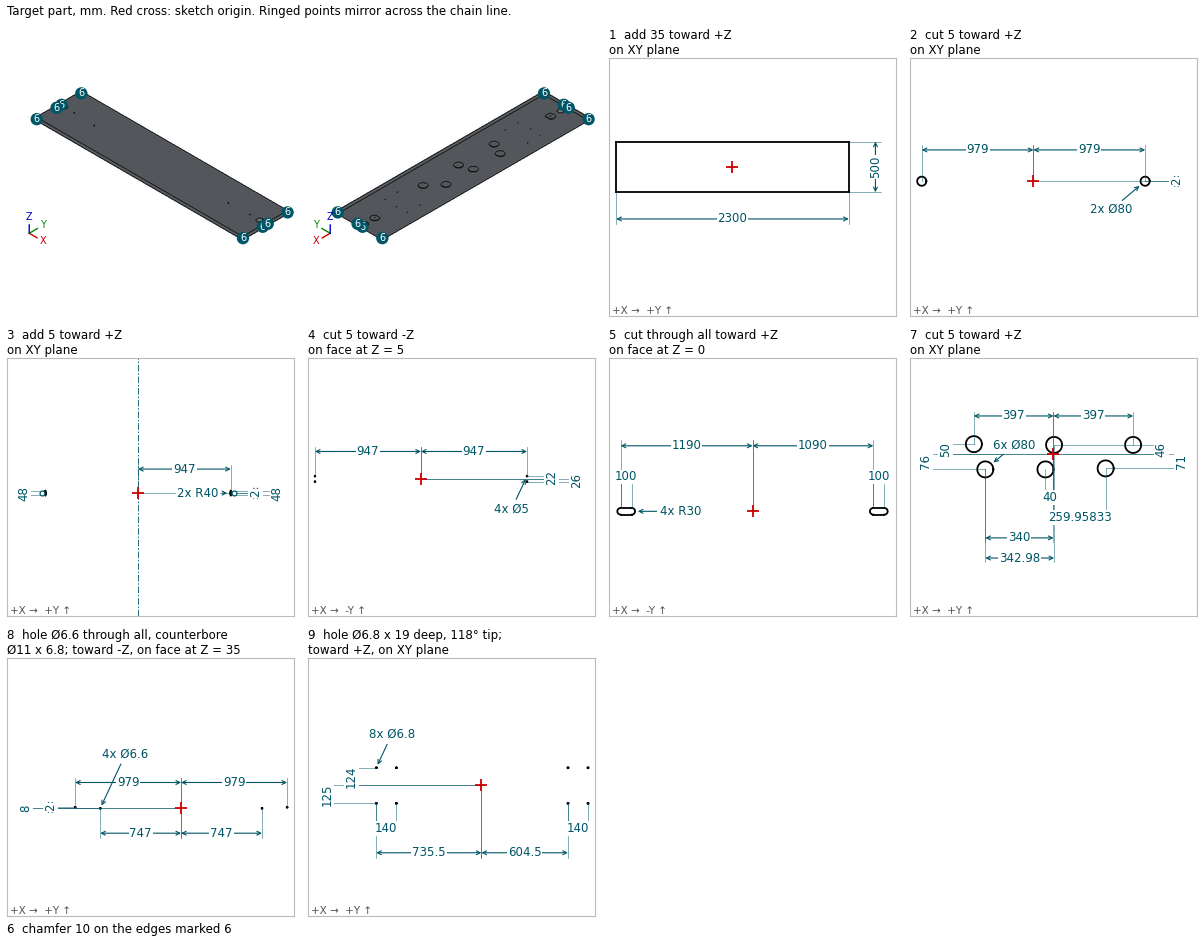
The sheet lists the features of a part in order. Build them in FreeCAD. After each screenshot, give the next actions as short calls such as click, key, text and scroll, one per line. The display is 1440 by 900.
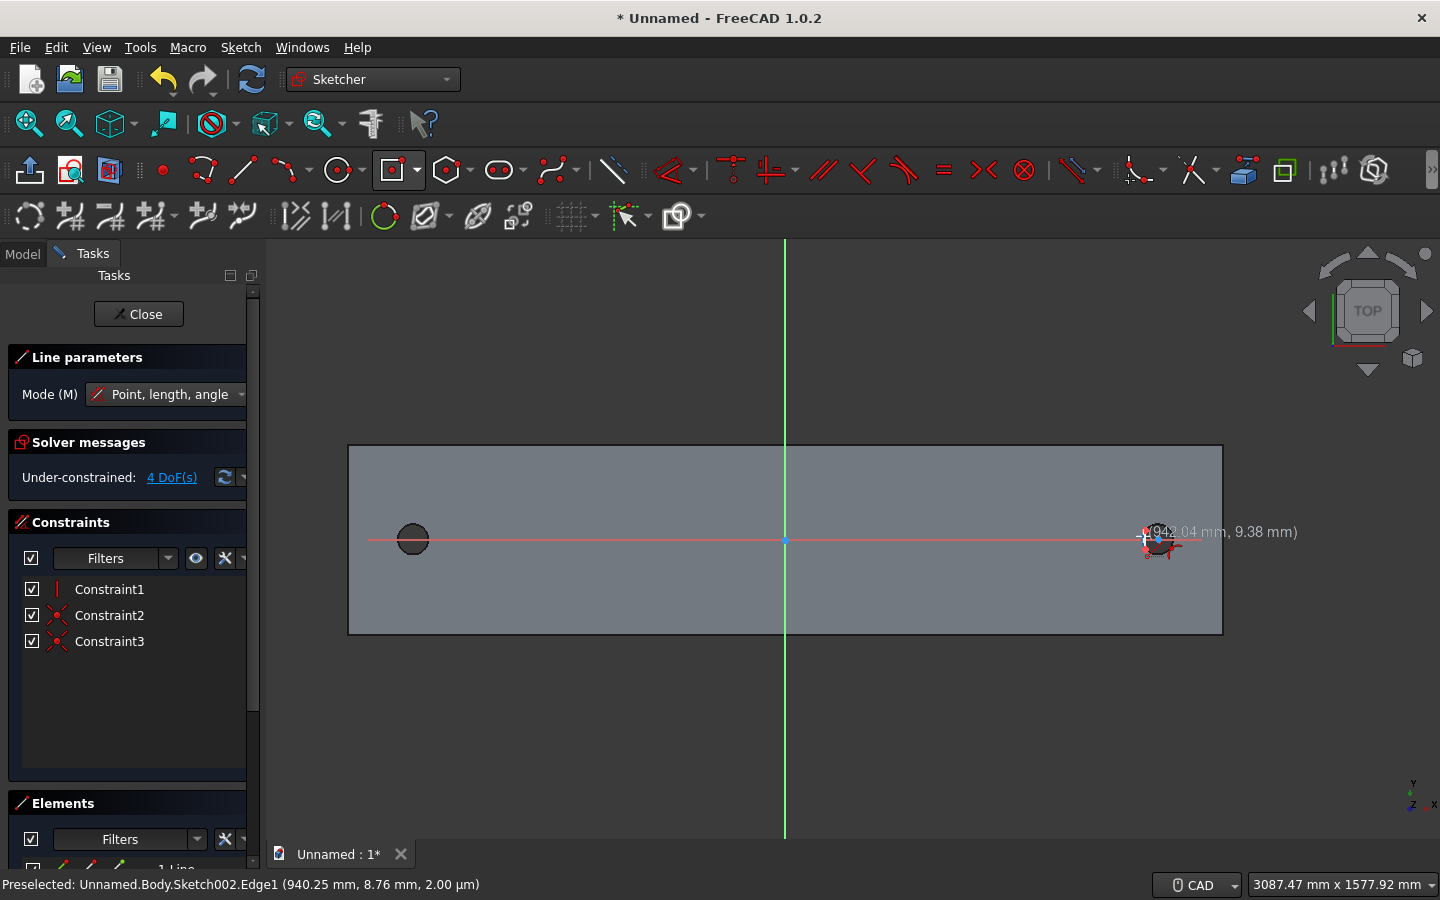
scroll(425, 549, up, 4)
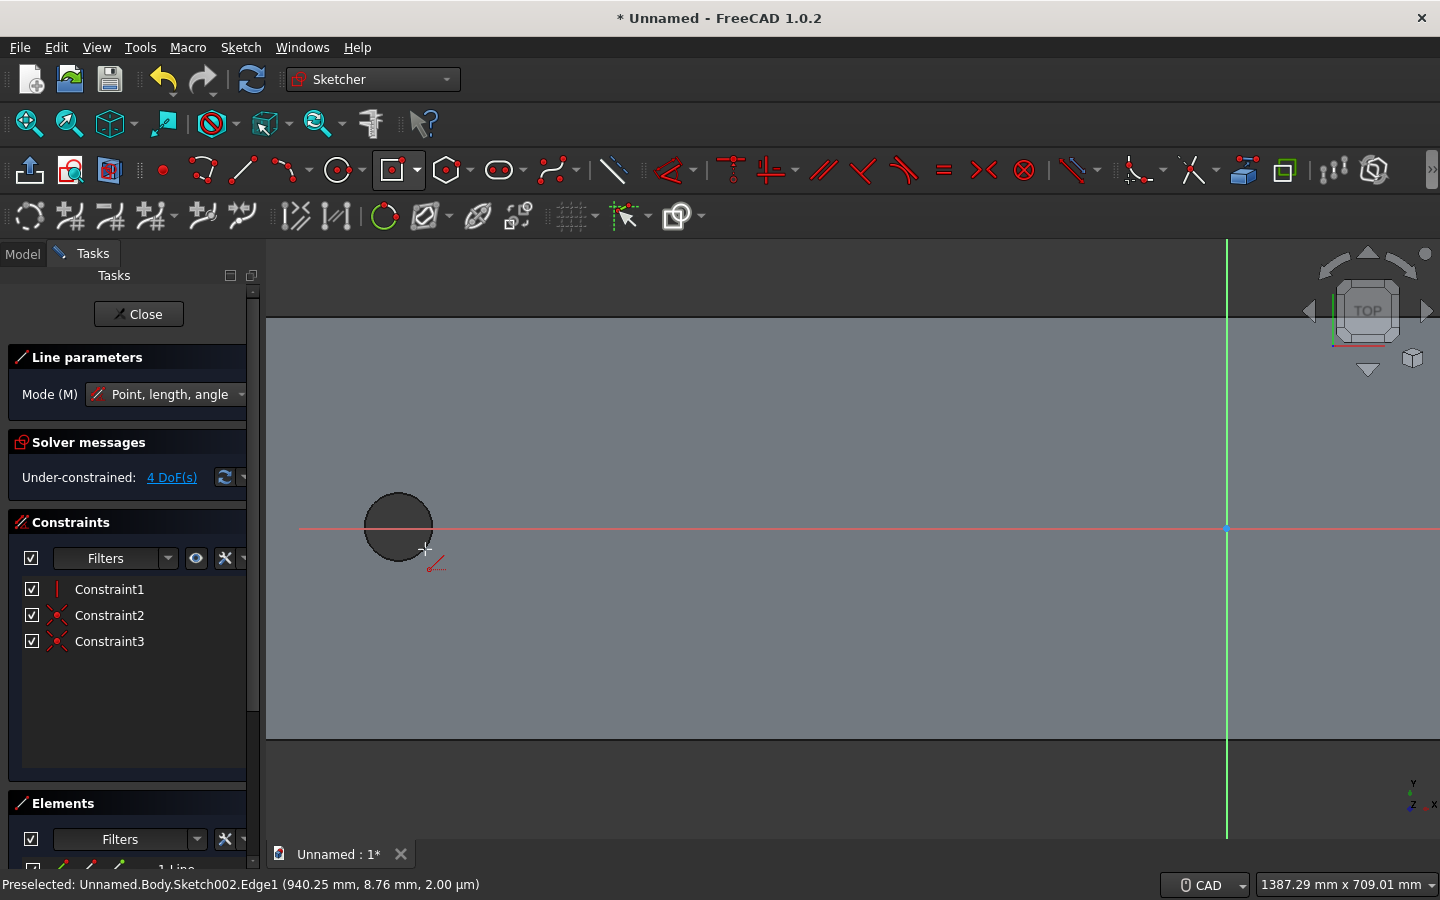
click(426, 547)
click(426, 507)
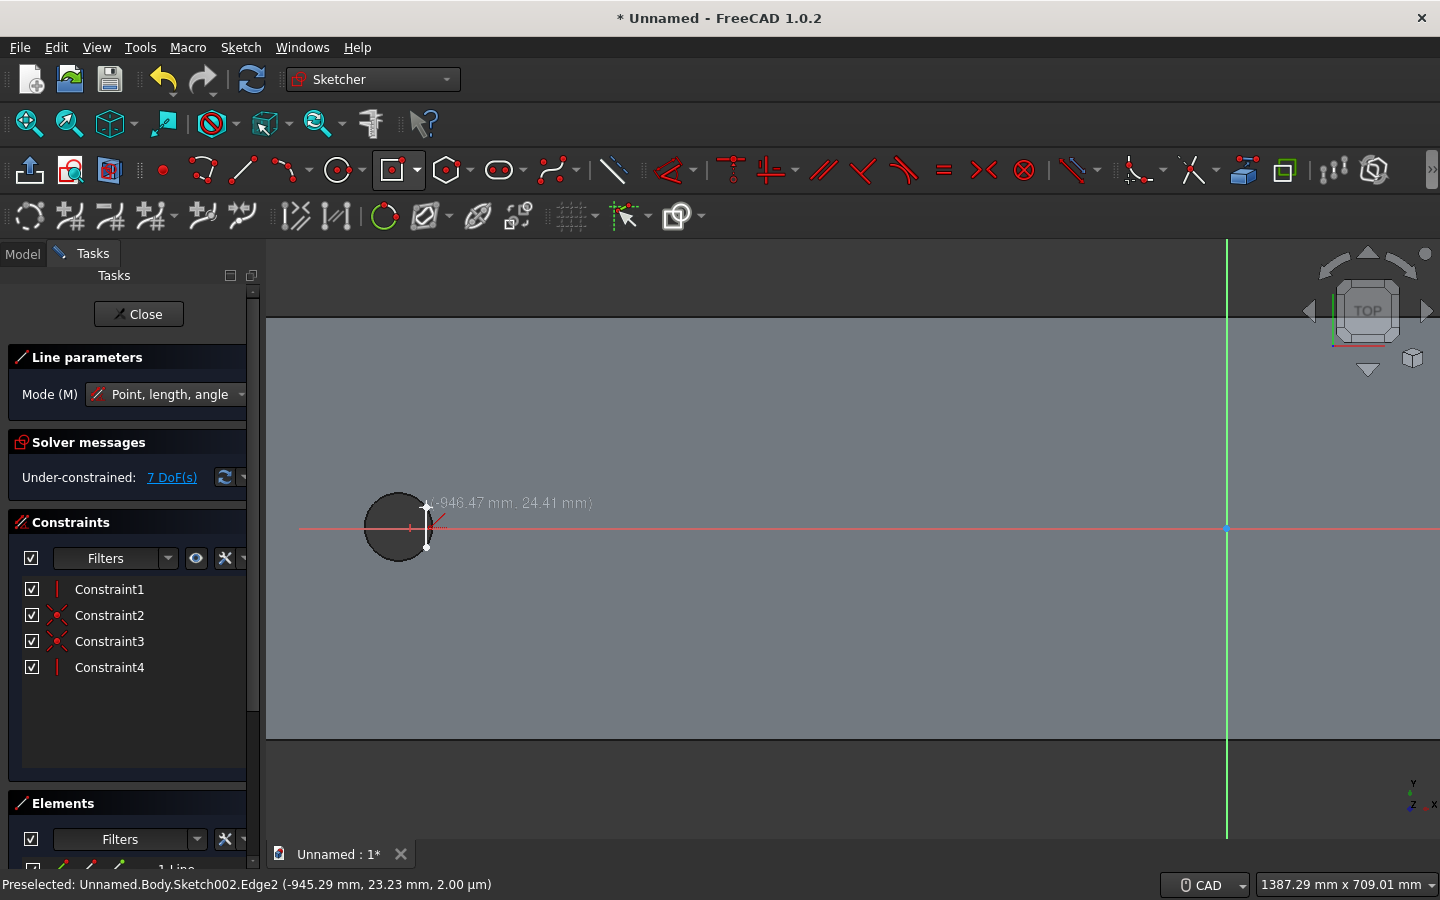
click(284, 170)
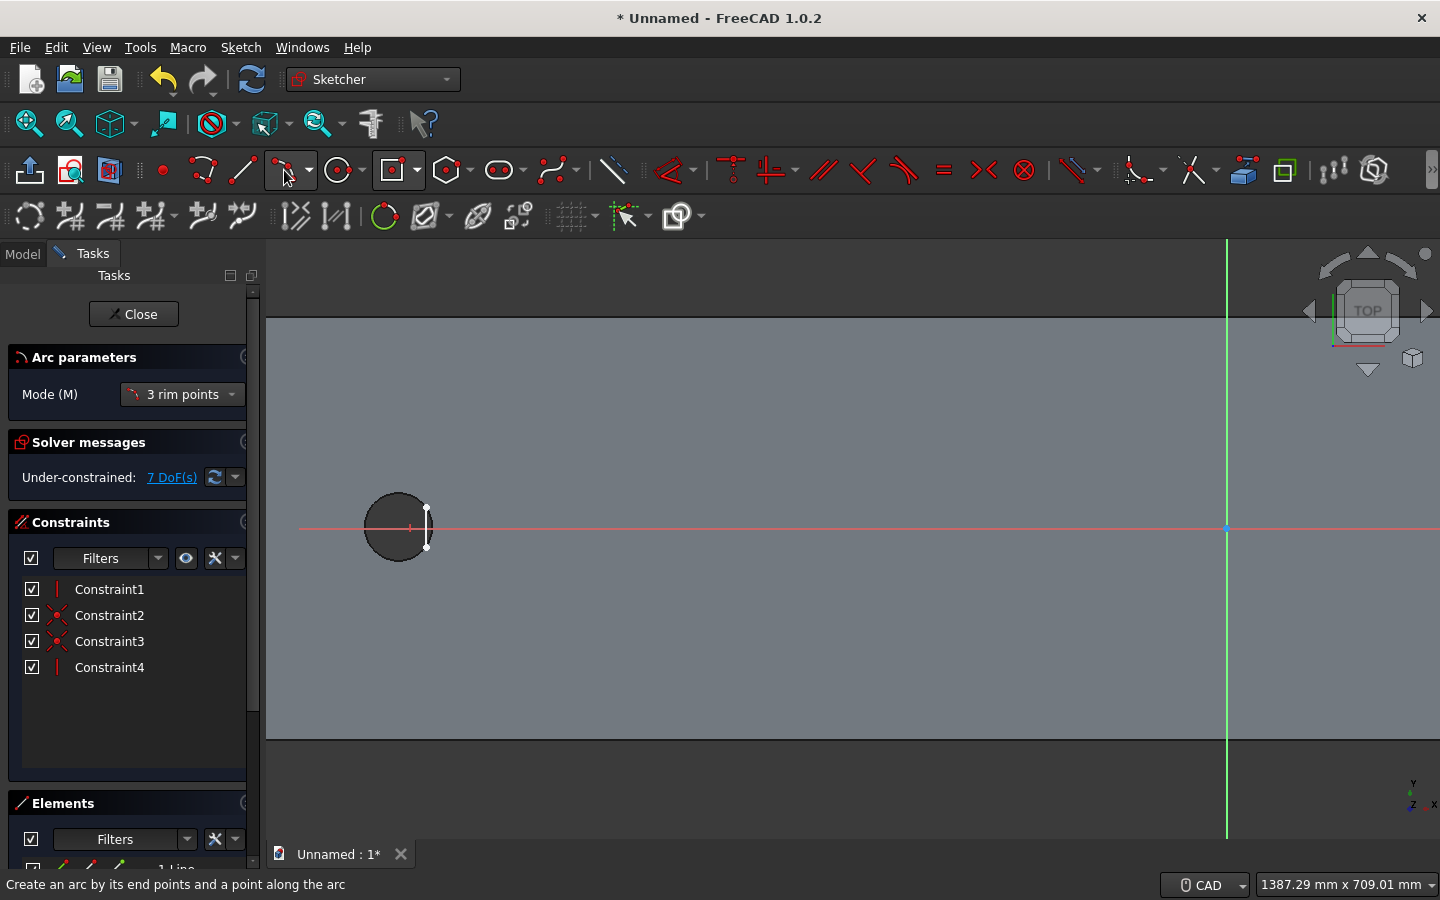
click(426, 508)
click(426, 548)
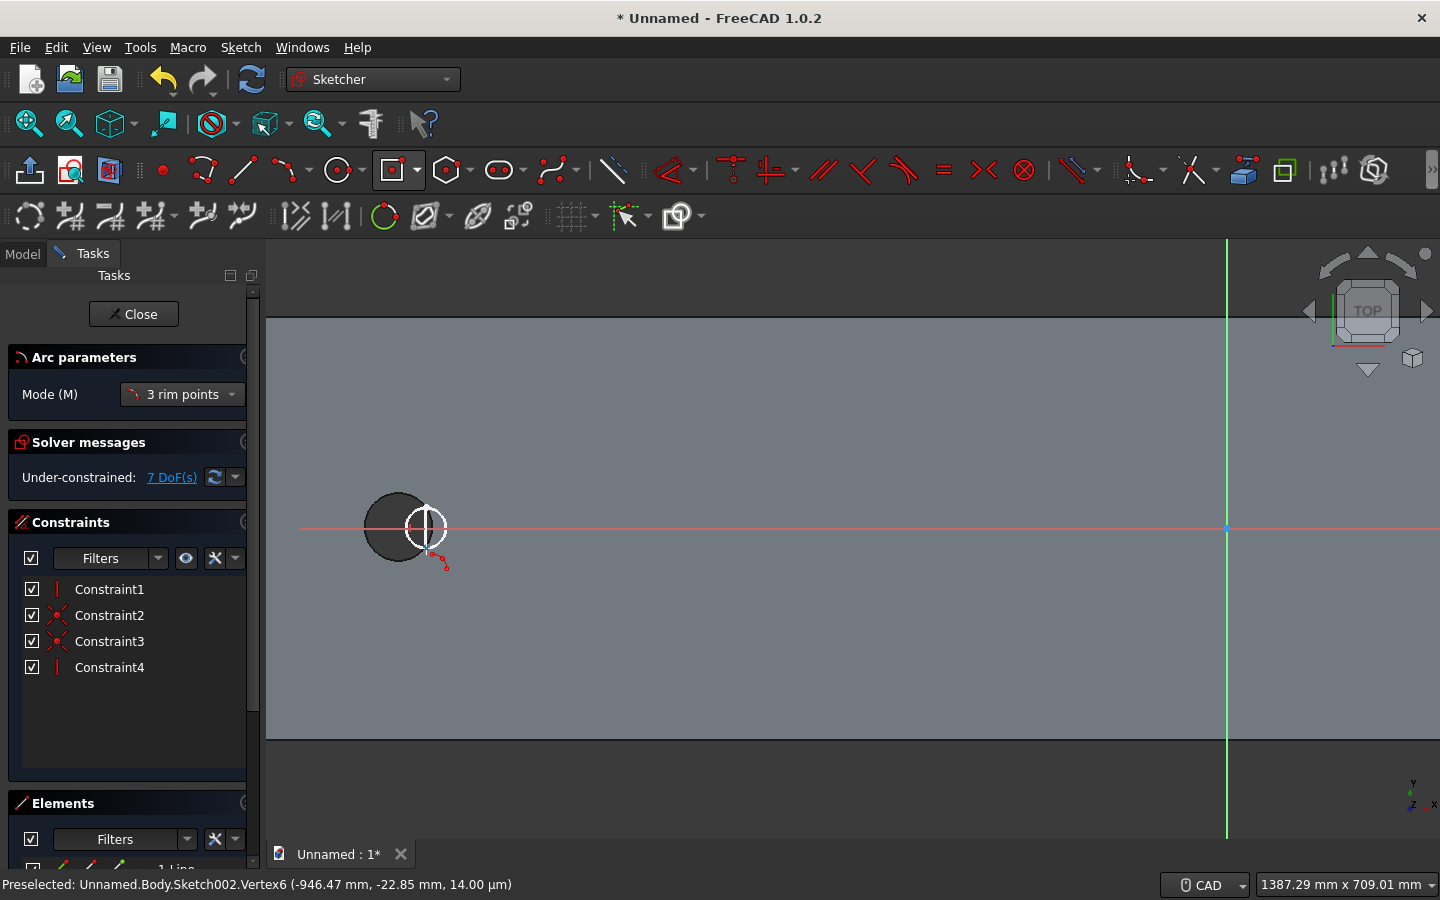
scroll(432, 523, up, 5)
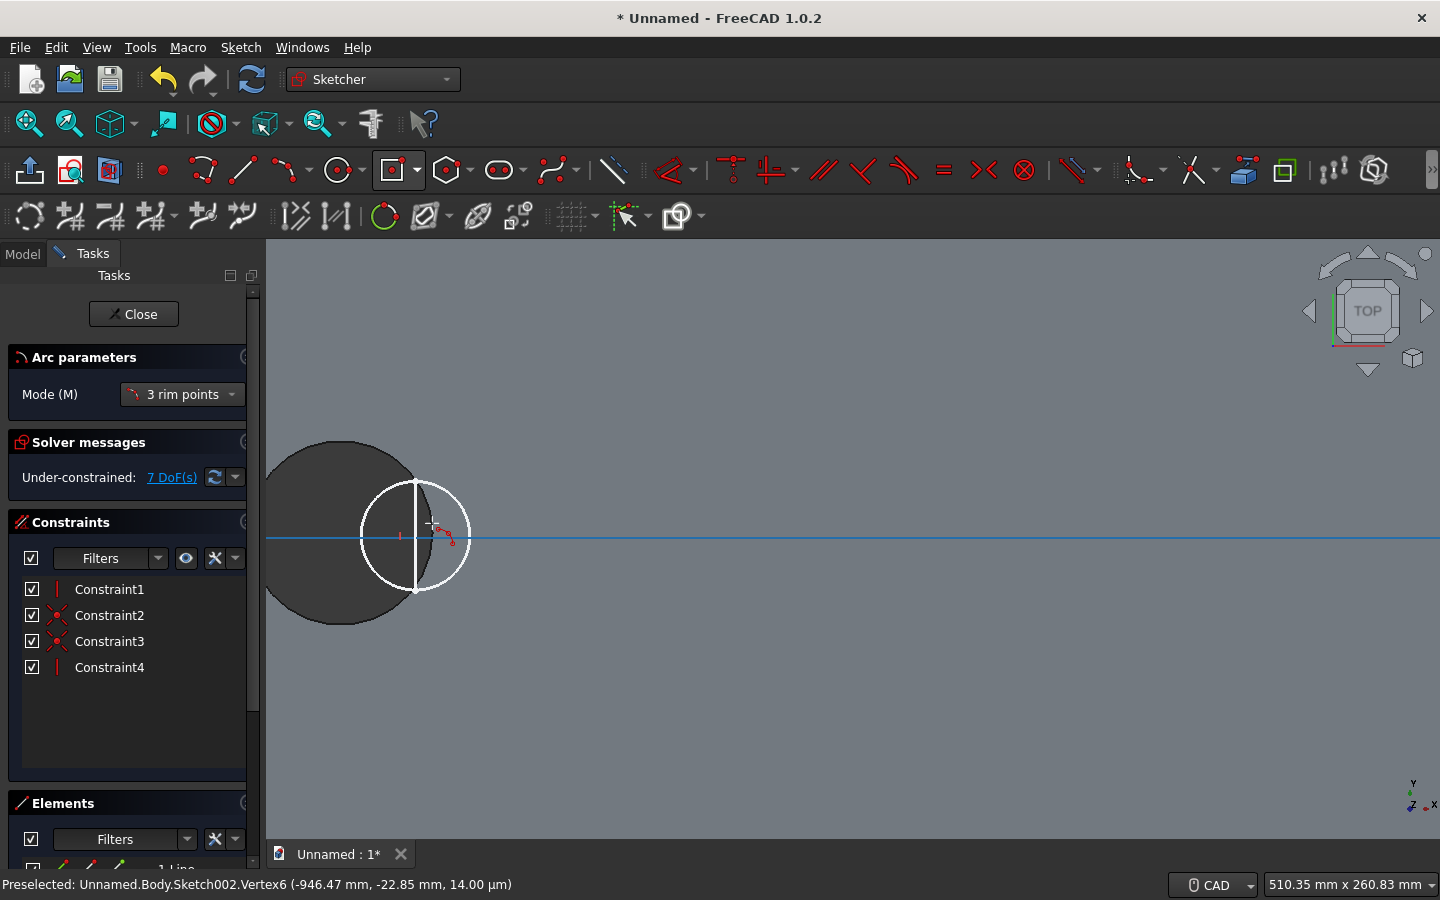
click(432, 521)
key(Escape)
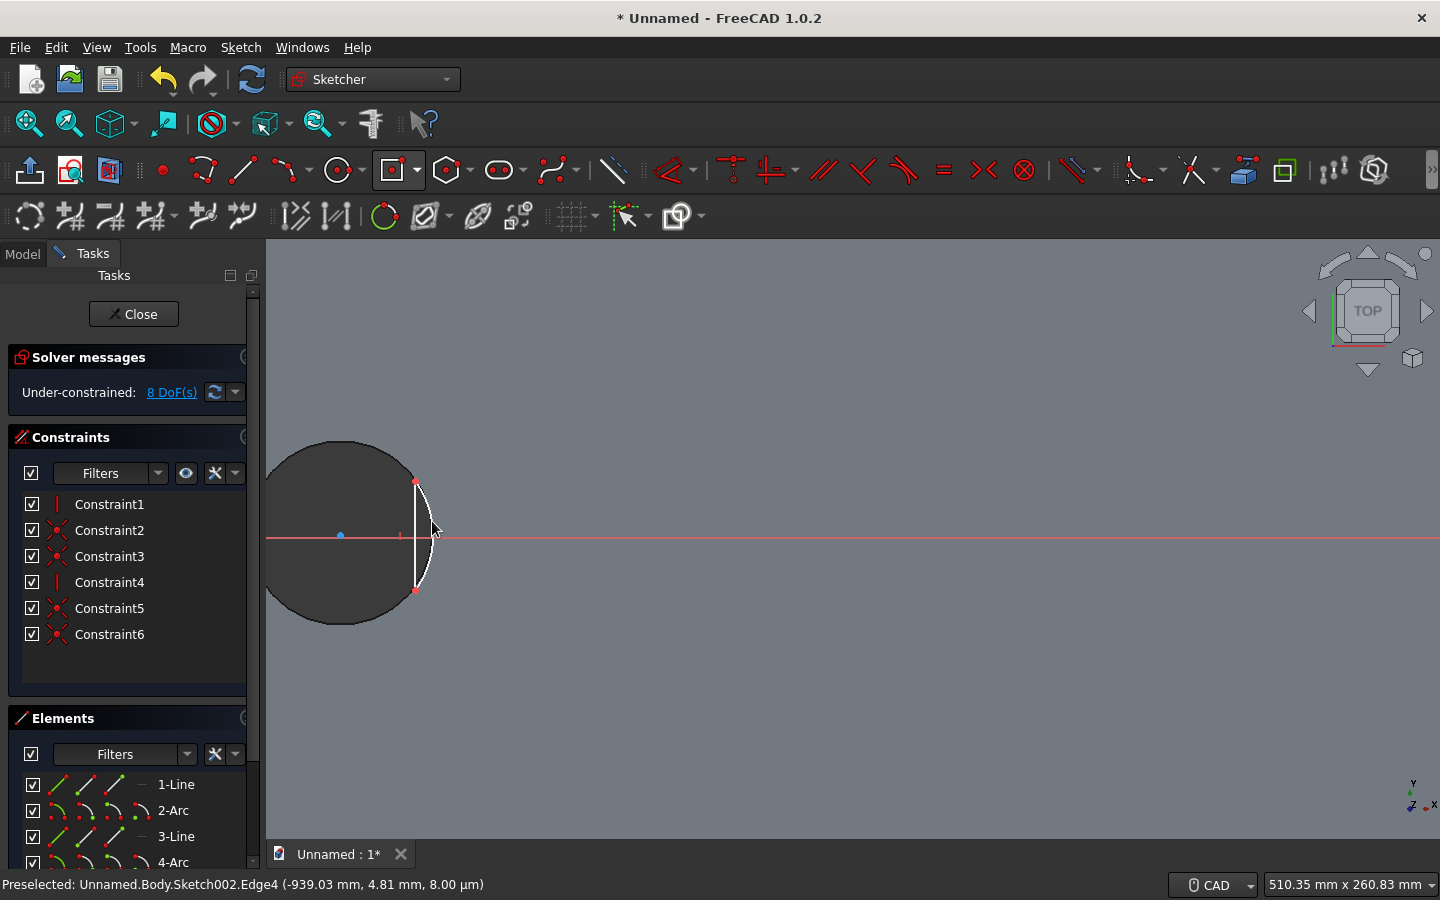
scroll(426, 540, down, 9)